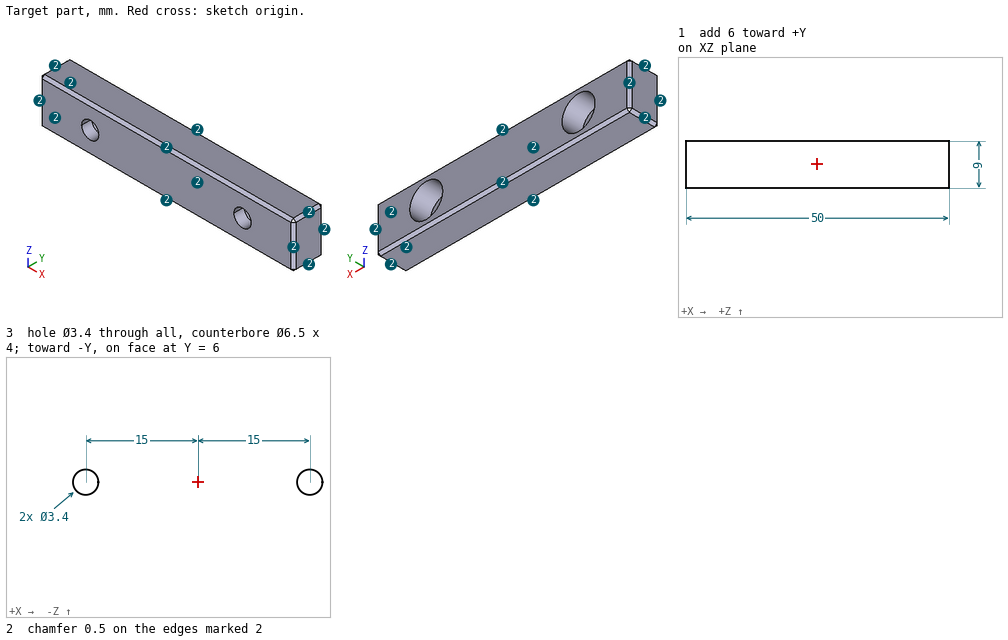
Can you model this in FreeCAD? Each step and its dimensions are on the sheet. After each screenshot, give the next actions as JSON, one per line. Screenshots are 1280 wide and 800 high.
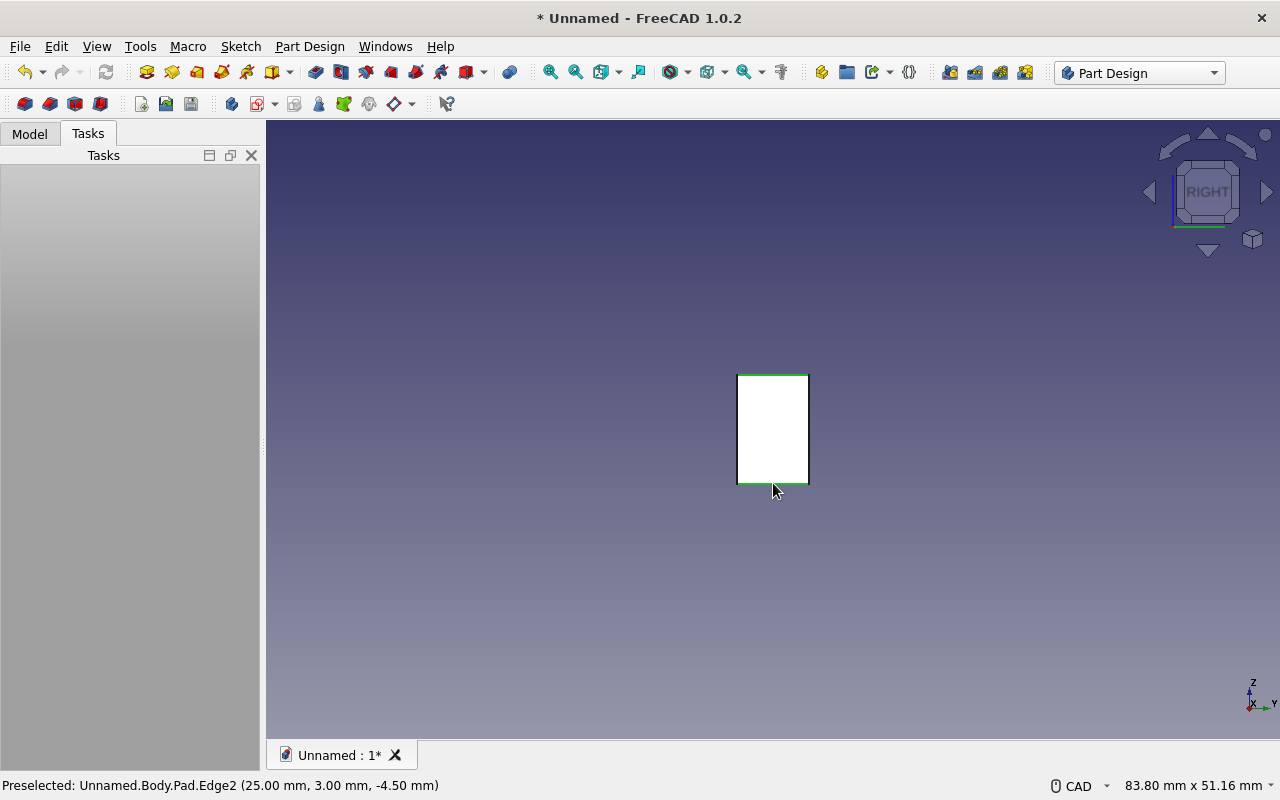
{"action": "key", "text": "5"}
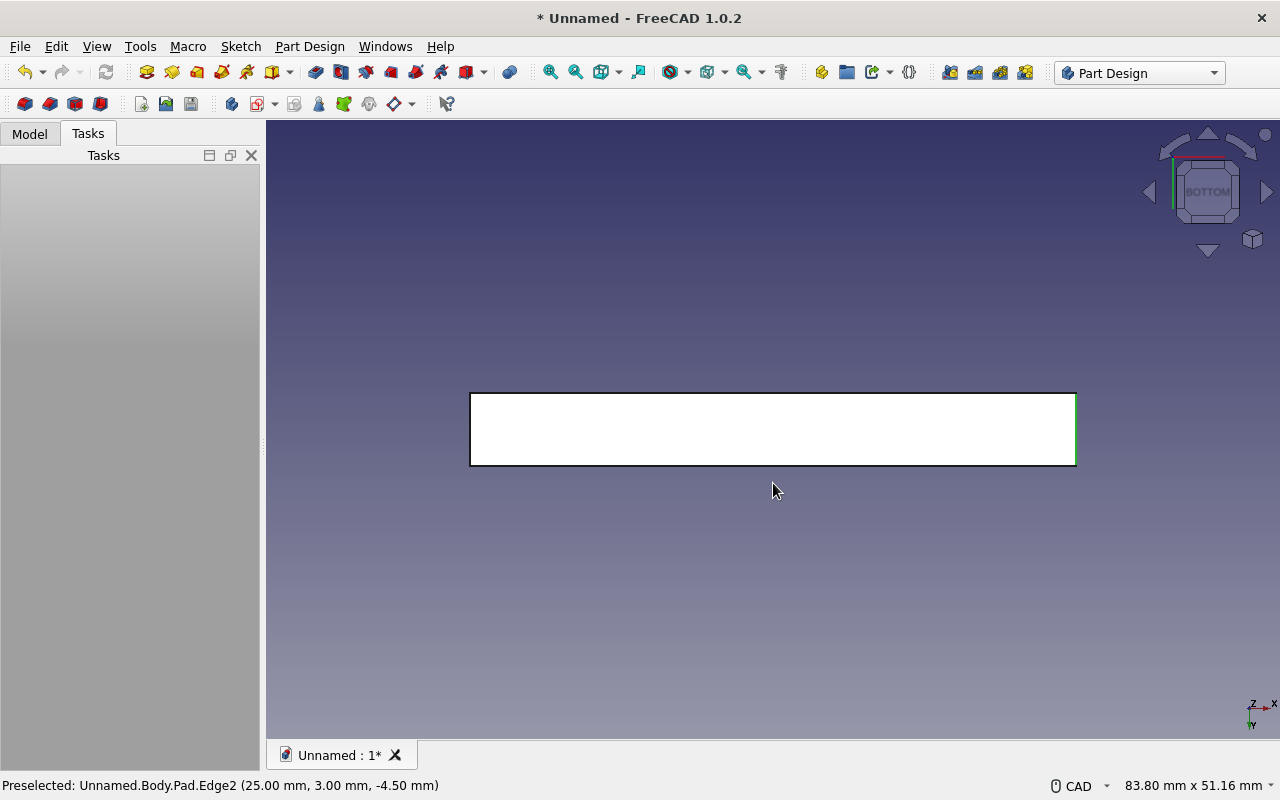
{"action": "left_click", "coordinate": [470, 428], "text": "ctrl"}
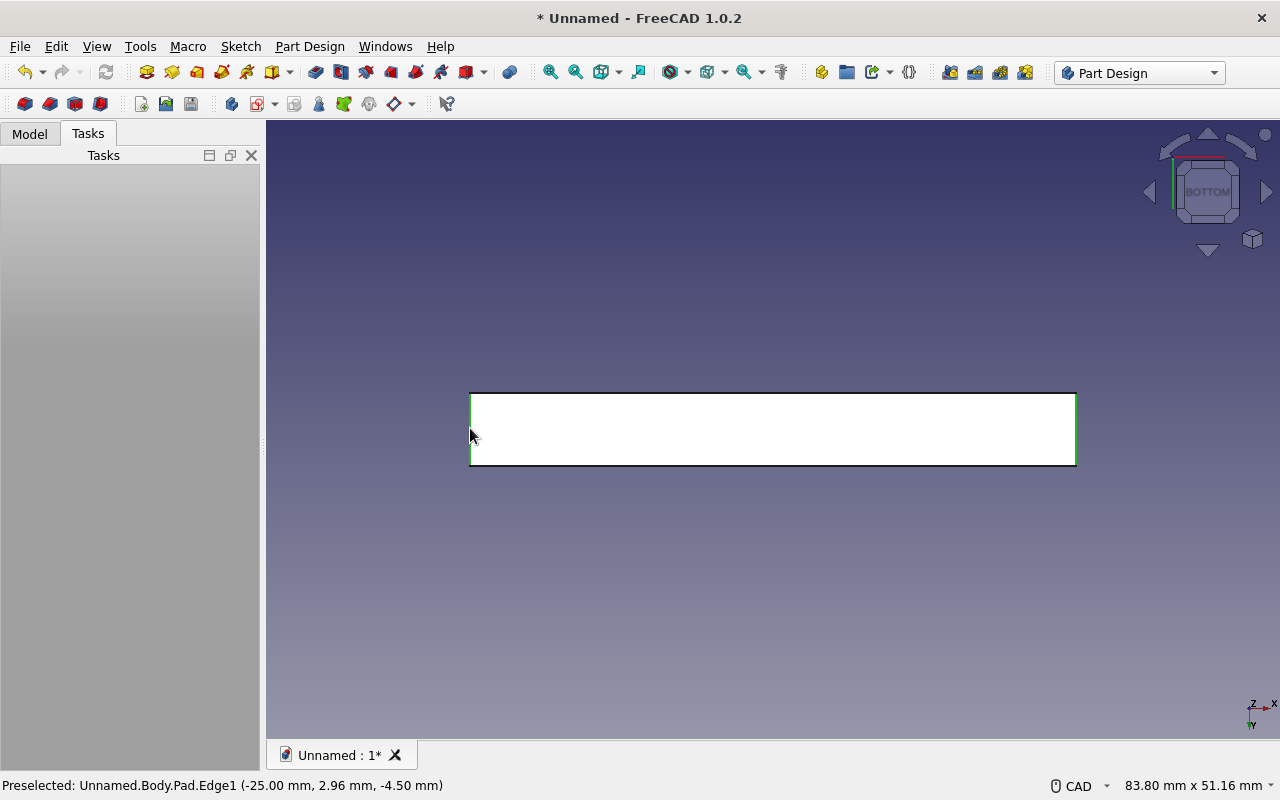
{"action": "key", "text": "4"}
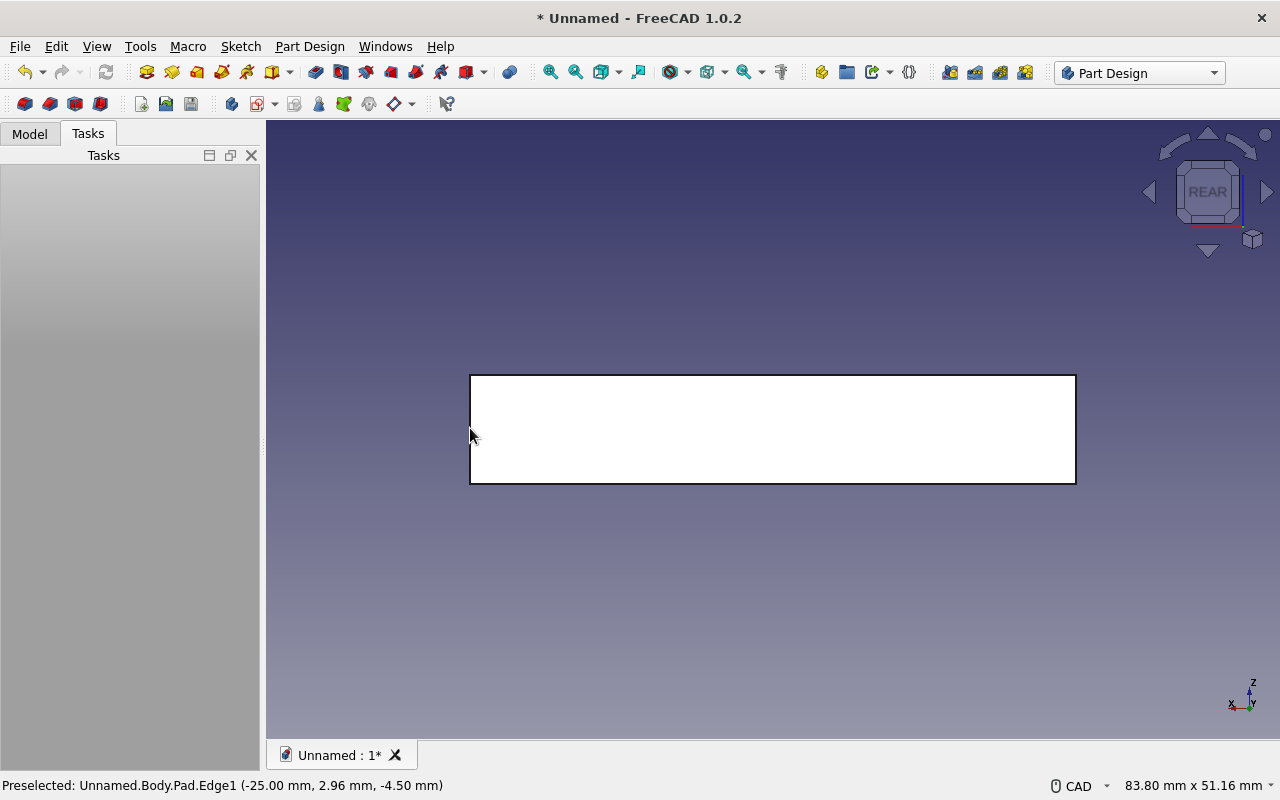
{"action": "left_click", "coordinate": [600, 429], "text": "ctrl"}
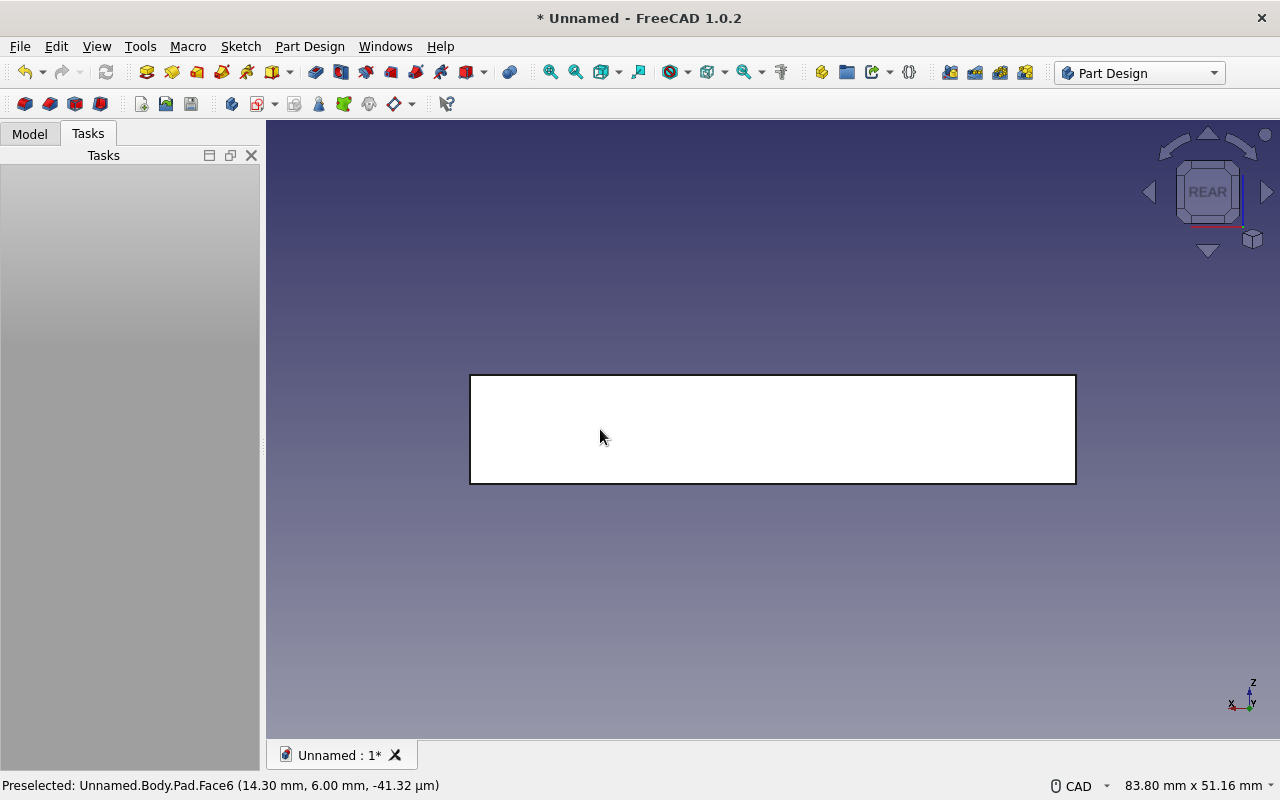
{"action": "left_click", "coordinate": [50, 104]}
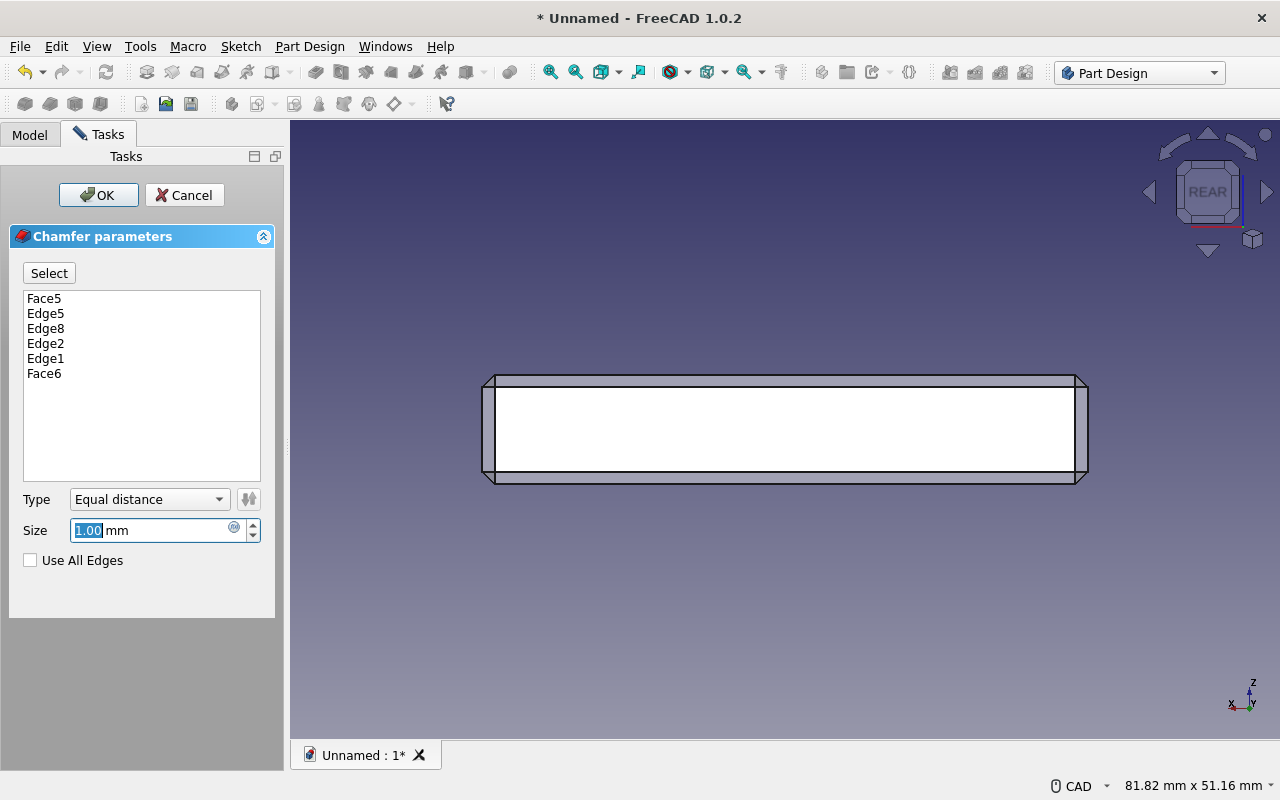
{"action": "type", "text": "0.5"}
{"action": "key", "text": "Tab"}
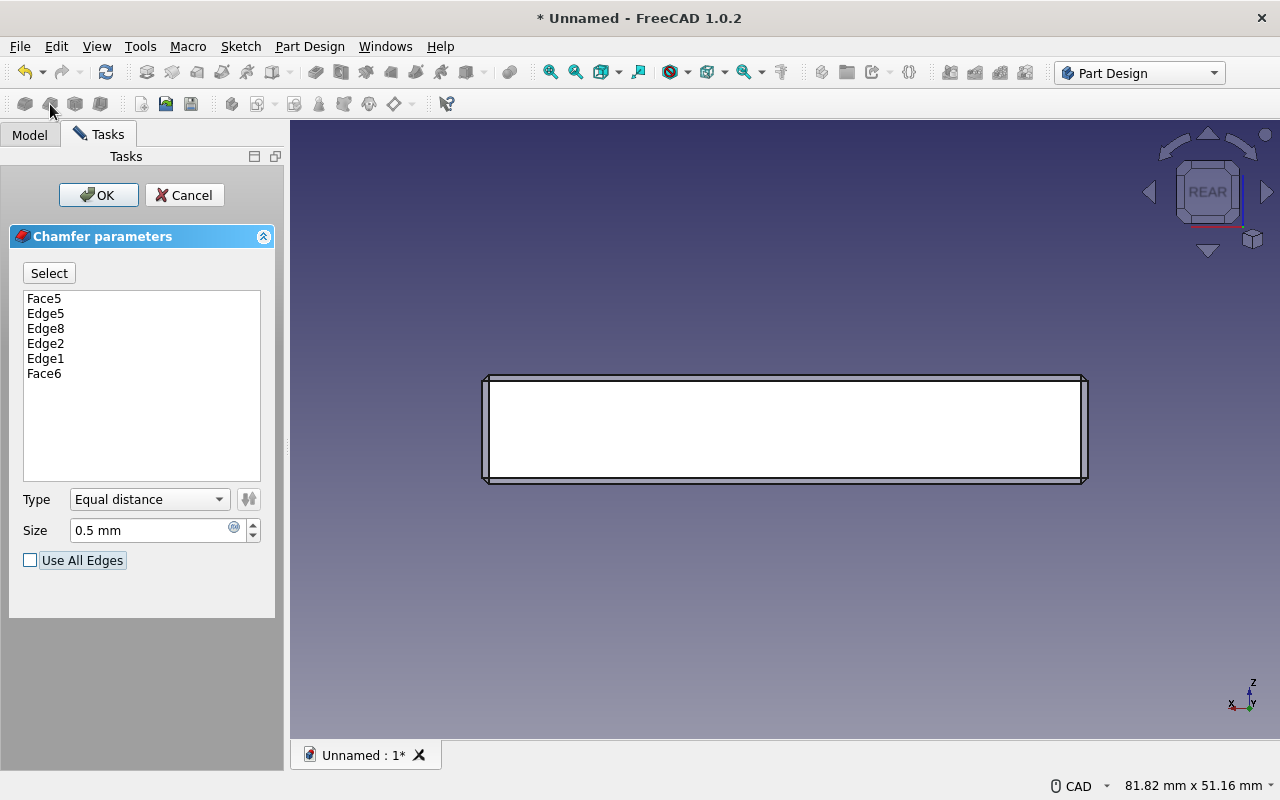
{"action": "left_click", "coordinate": [99, 195]}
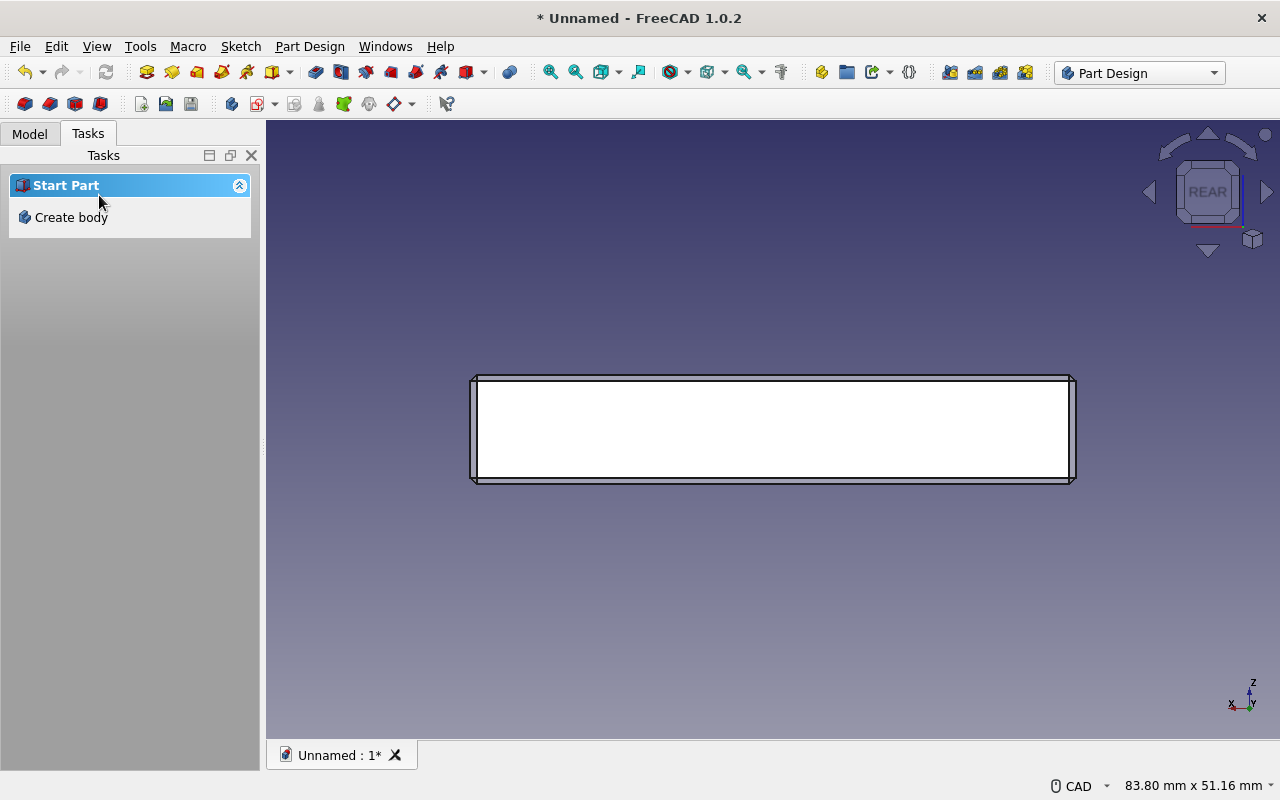
{"action": "left_click", "coordinate": [604, 429]}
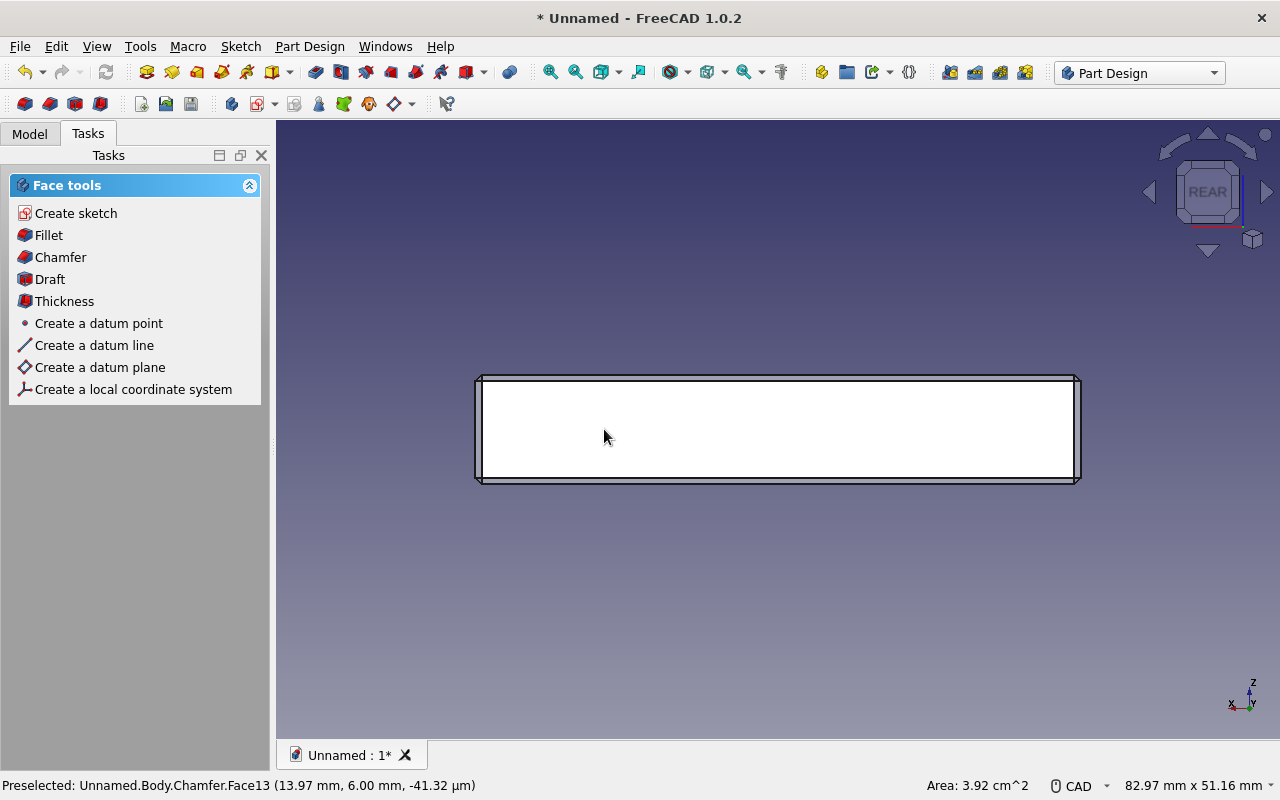
{"action": "left_click", "coordinate": [256, 104]}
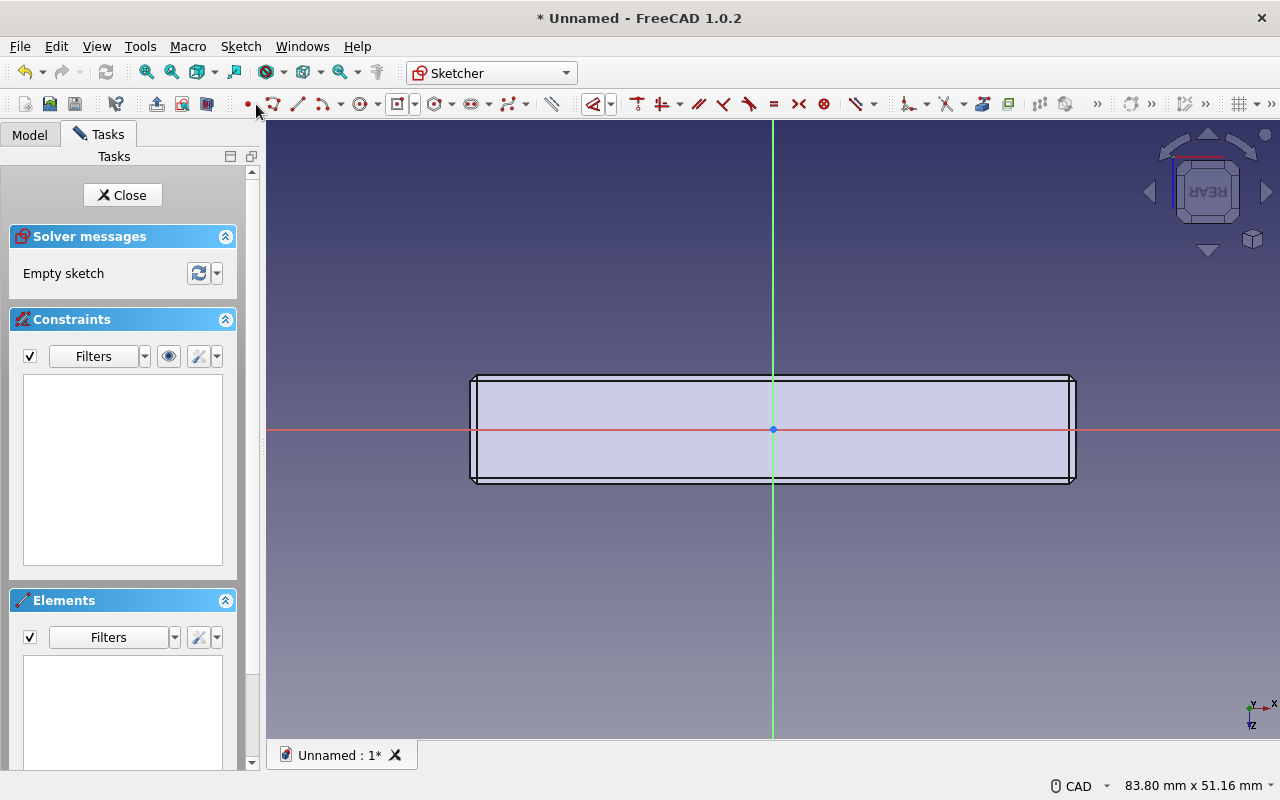
{"action": "scroll", "coordinate": [912, 429], "scroll_direction": "up", "scroll_amount": 2}